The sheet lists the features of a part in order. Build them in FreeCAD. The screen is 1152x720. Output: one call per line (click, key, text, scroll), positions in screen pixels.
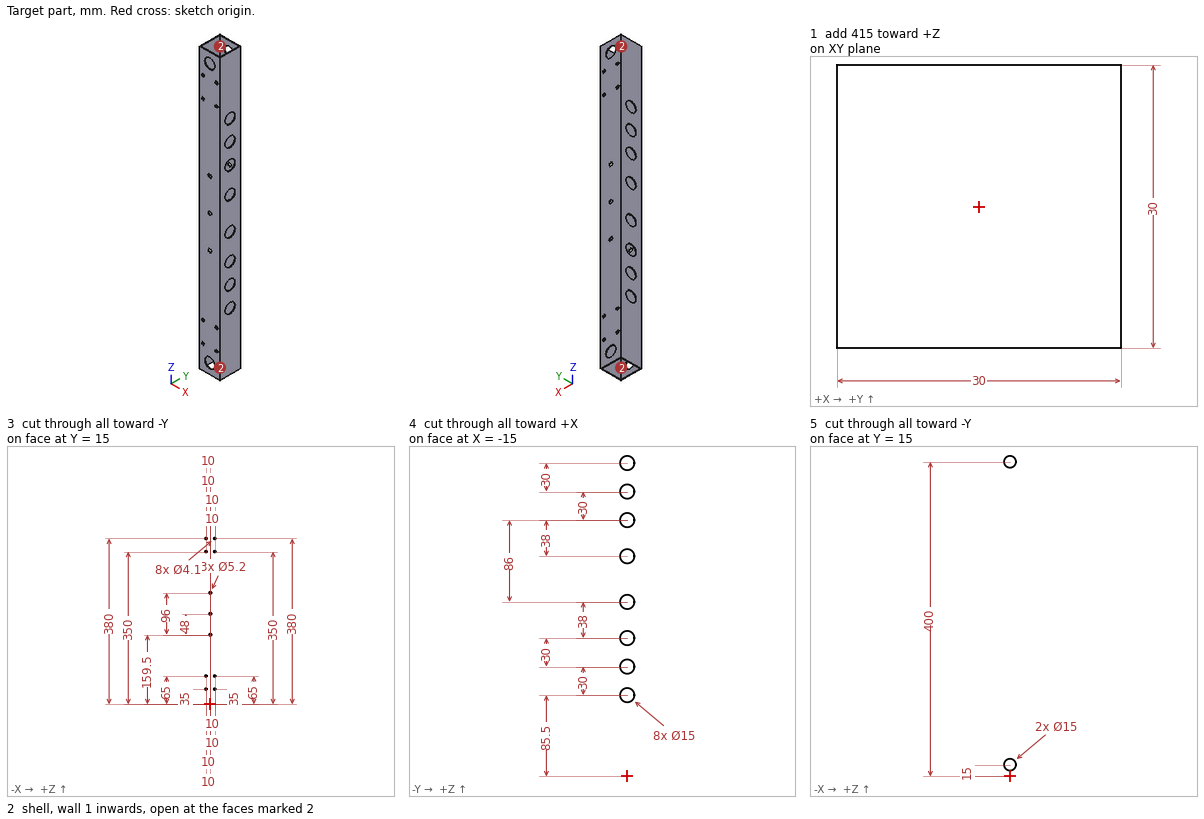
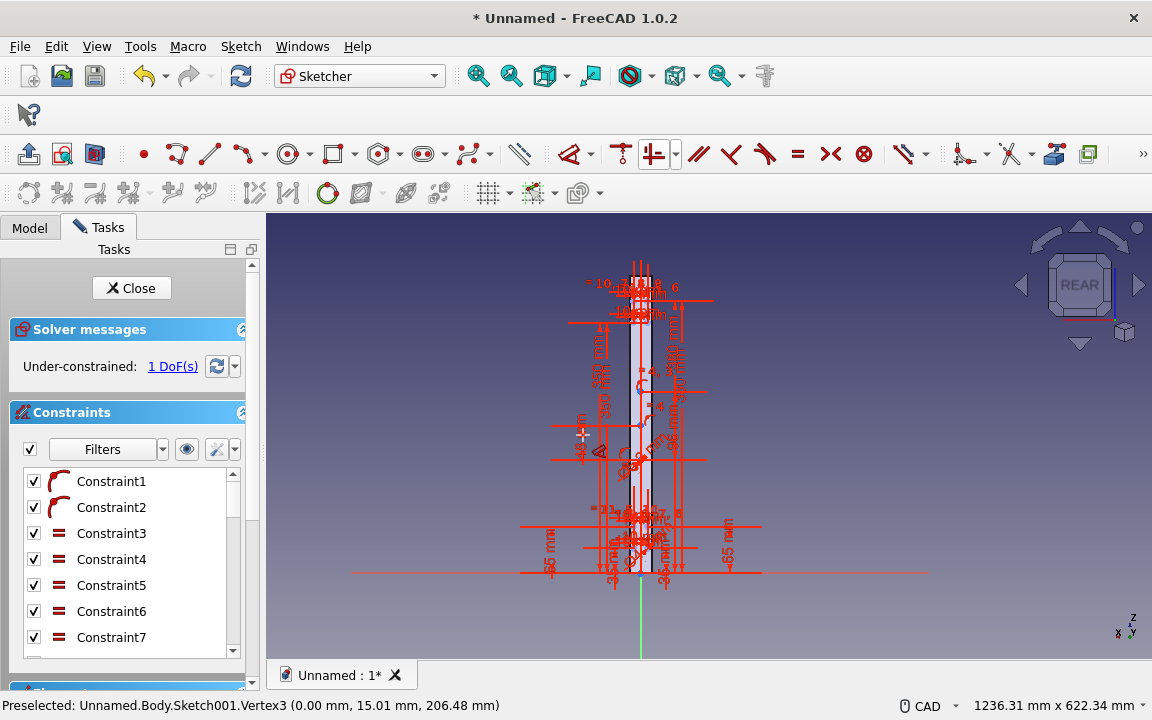
click(641, 460)
click(675, 491)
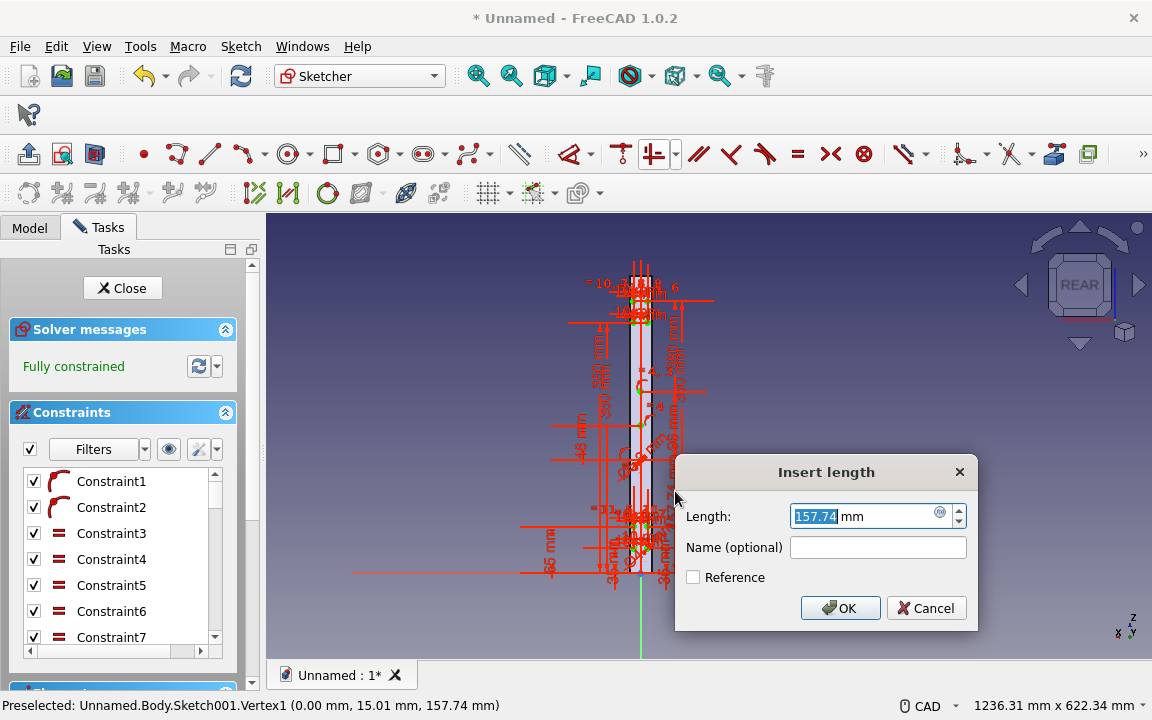
text(159.5)
key(Return)
key(Escape)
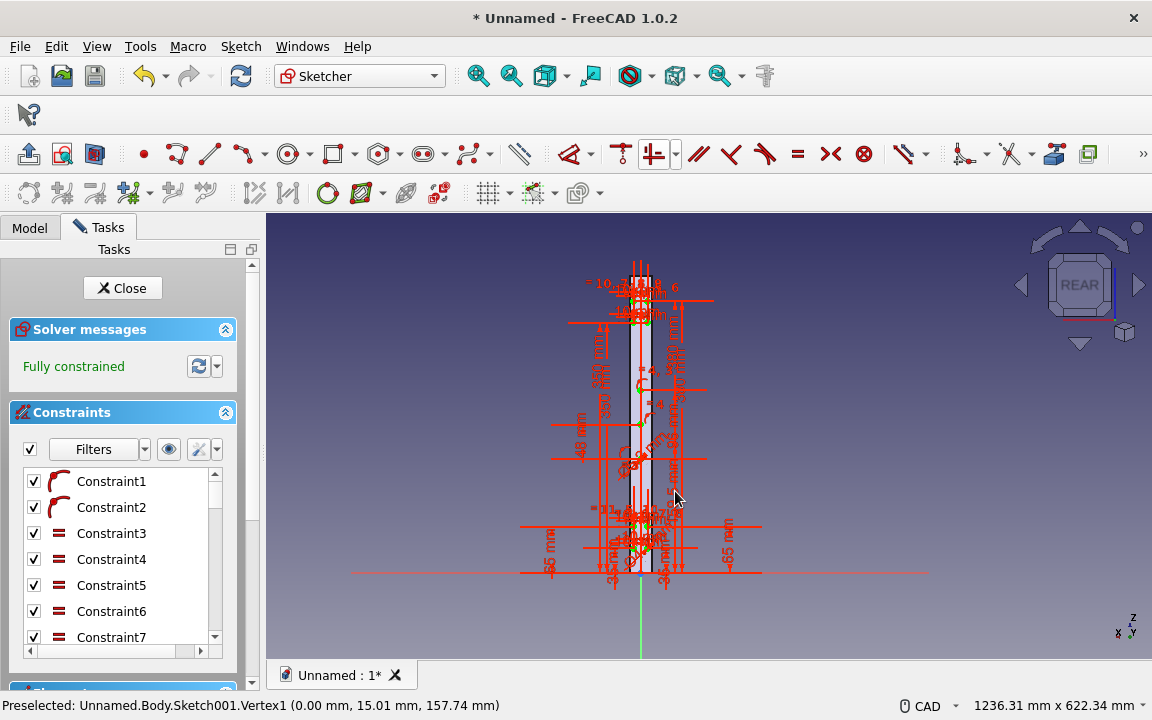
click(123, 288)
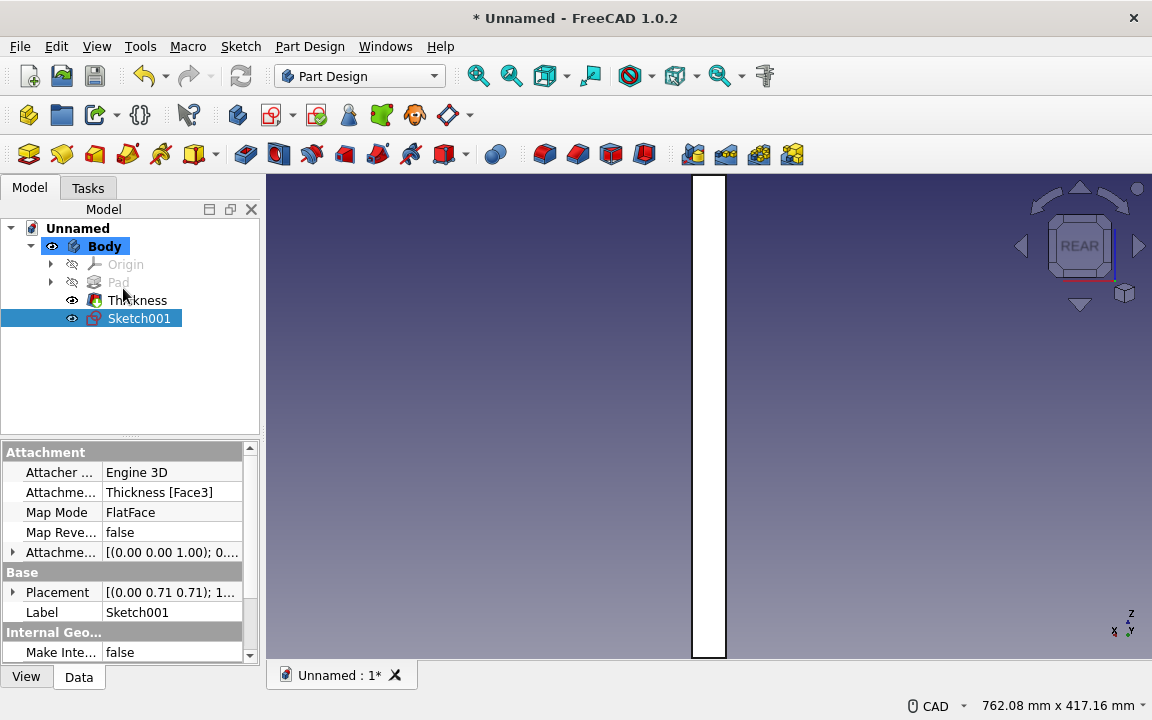
click(246, 154)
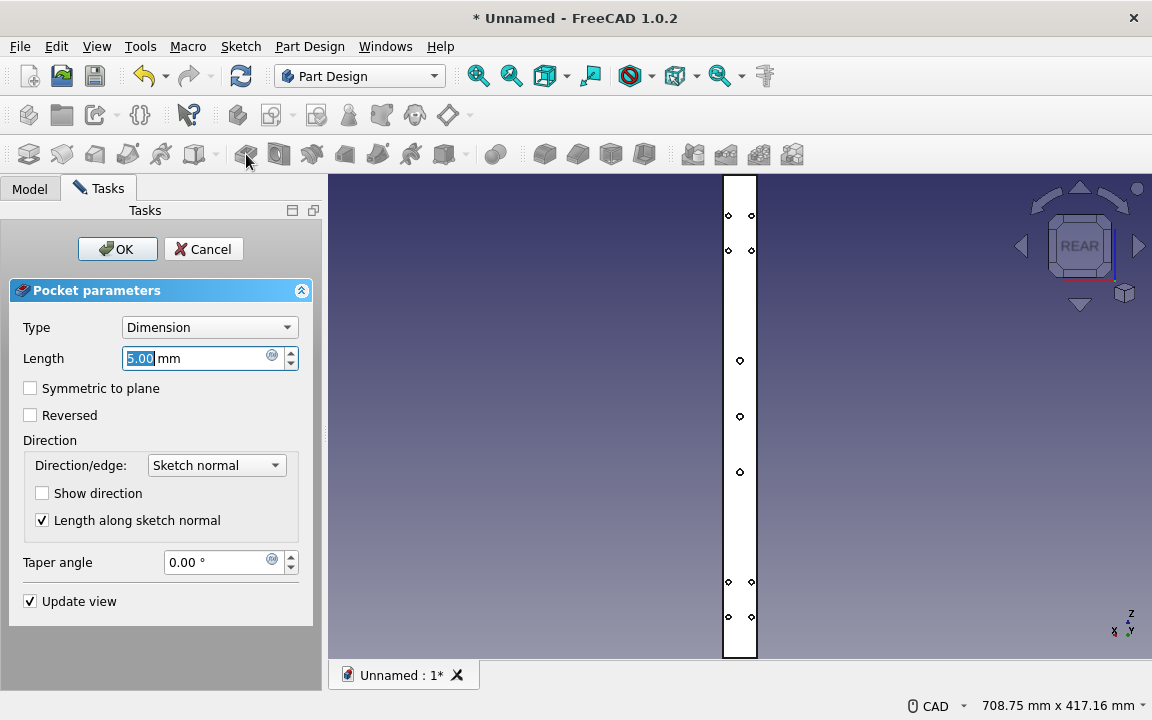
click(210, 328)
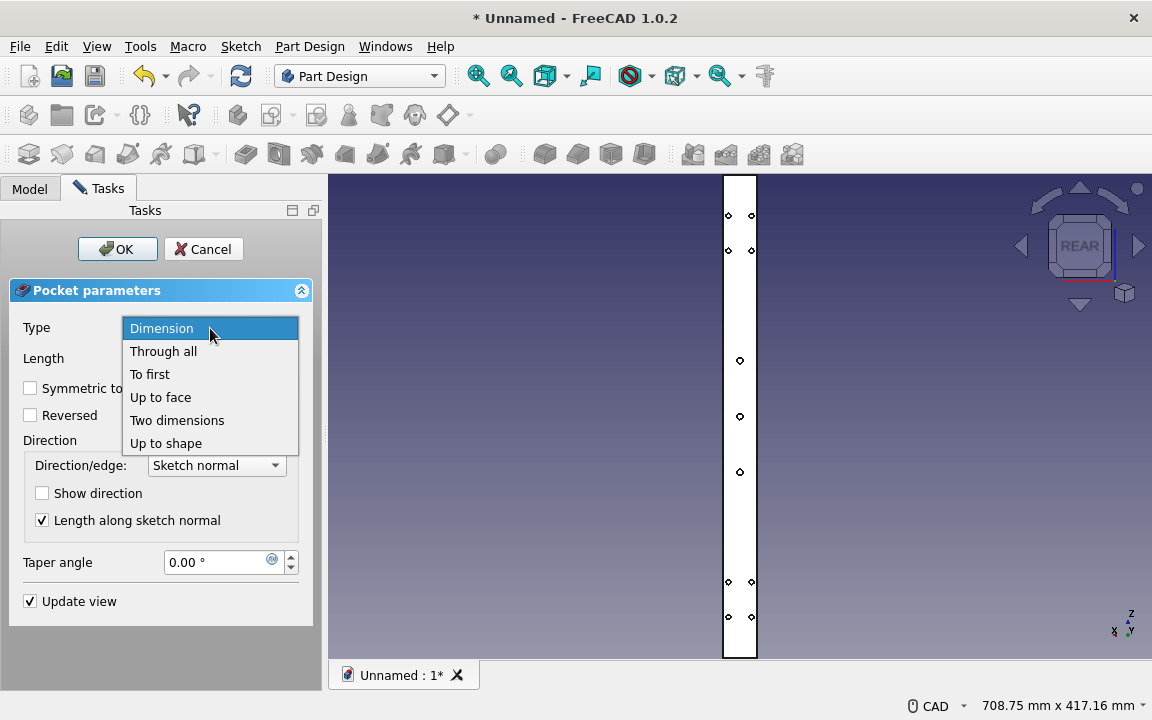
click(208, 352)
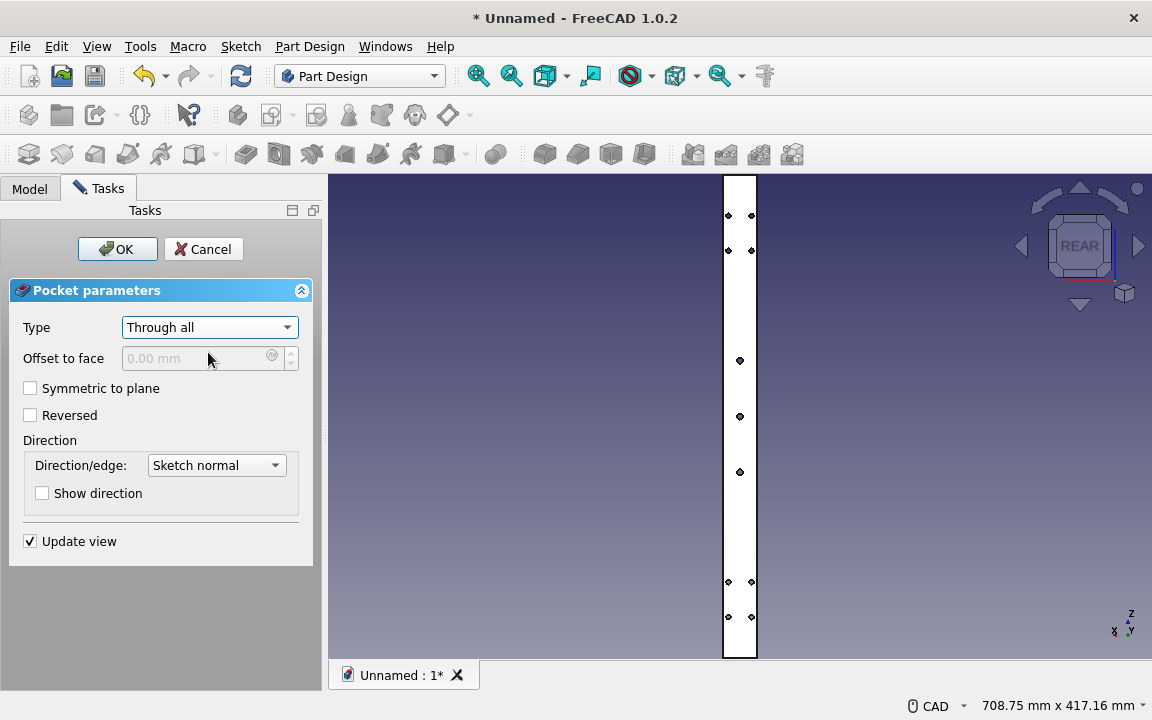
click(118, 249)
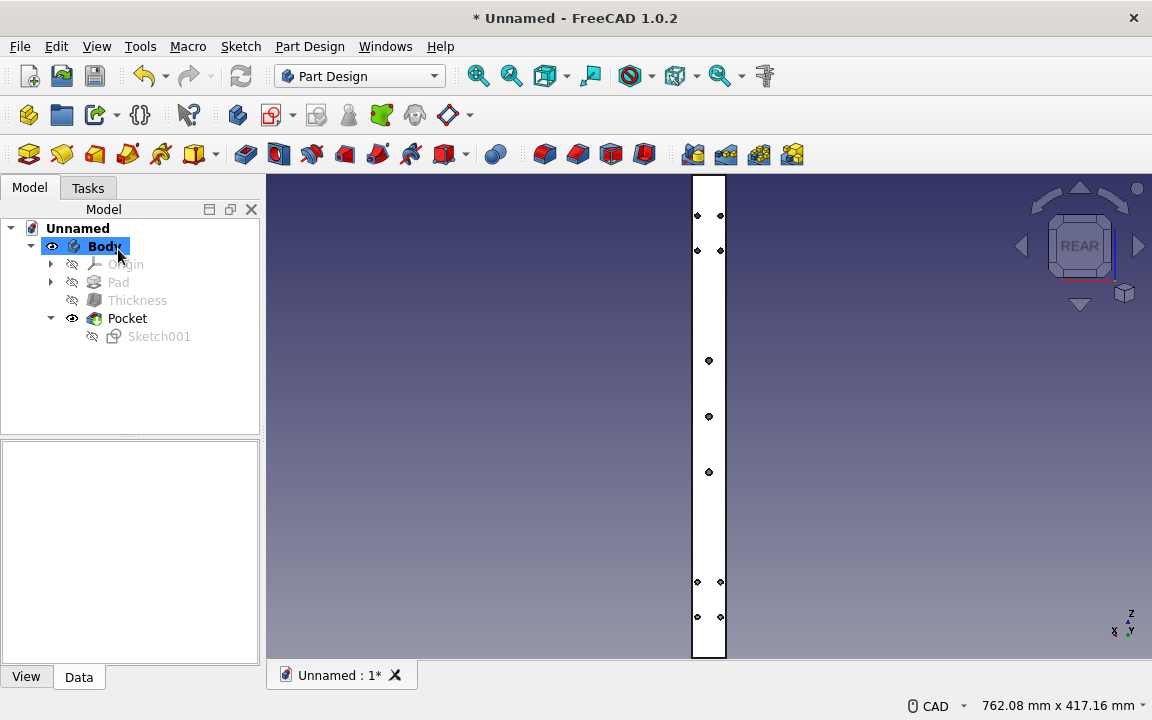
key(6)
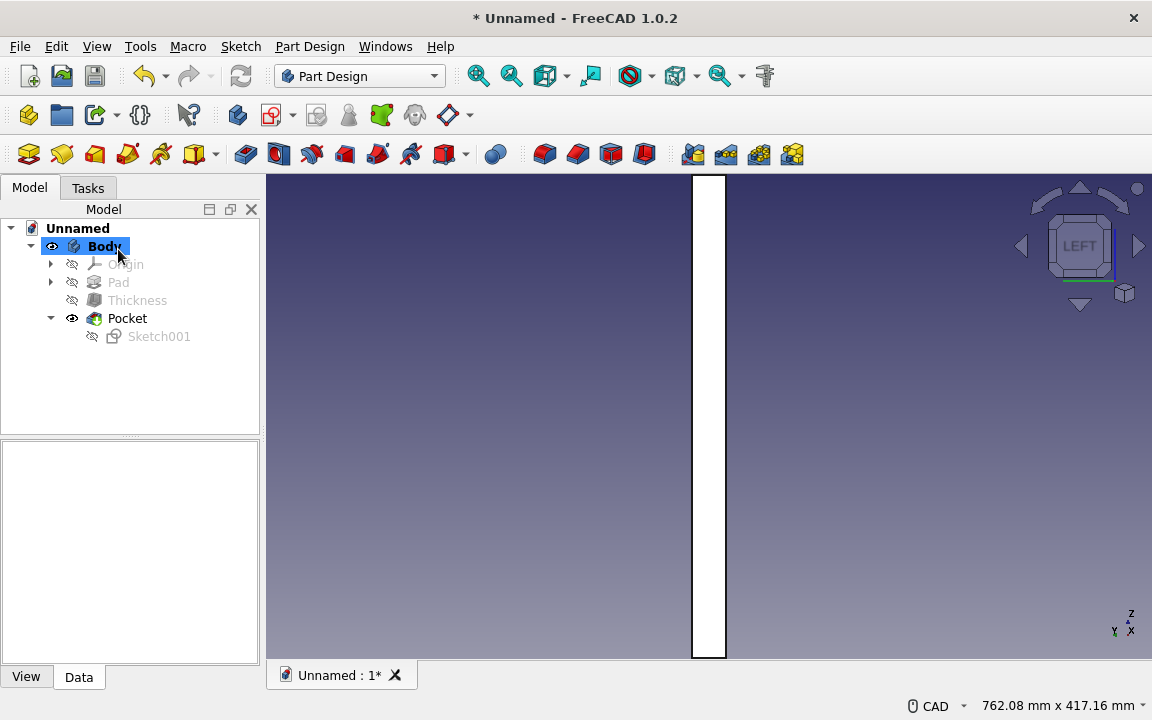
click(709, 209)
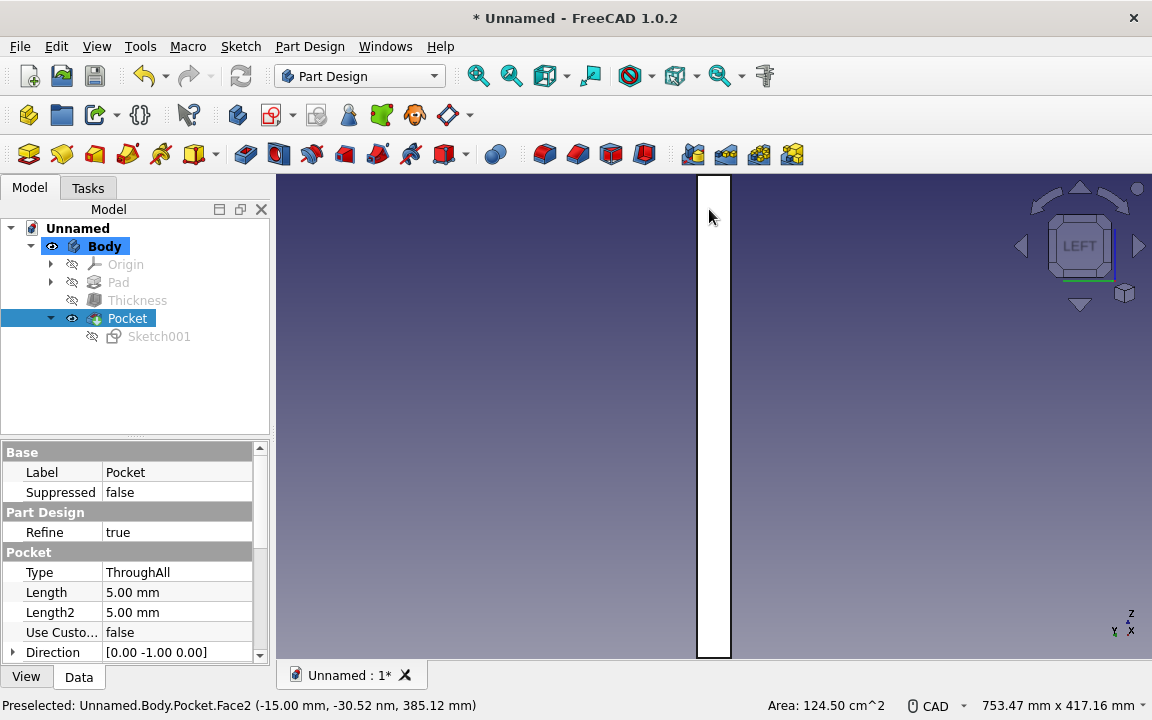
click(270, 116)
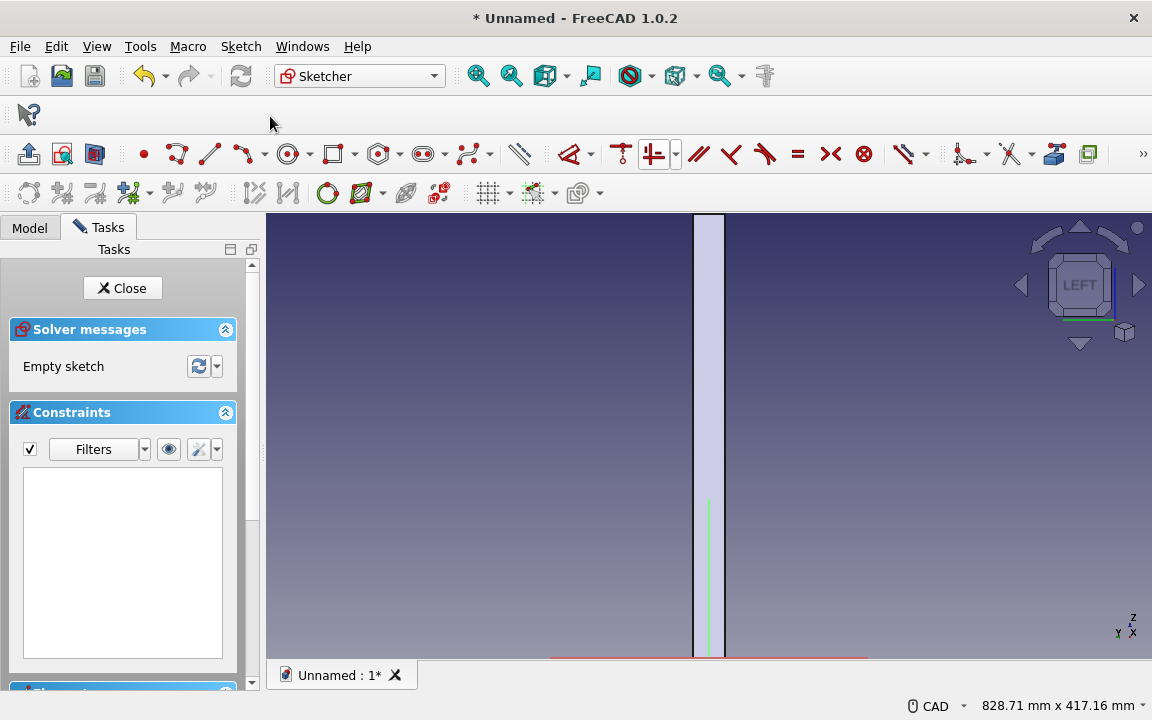
scroll(331, 248, down, 1)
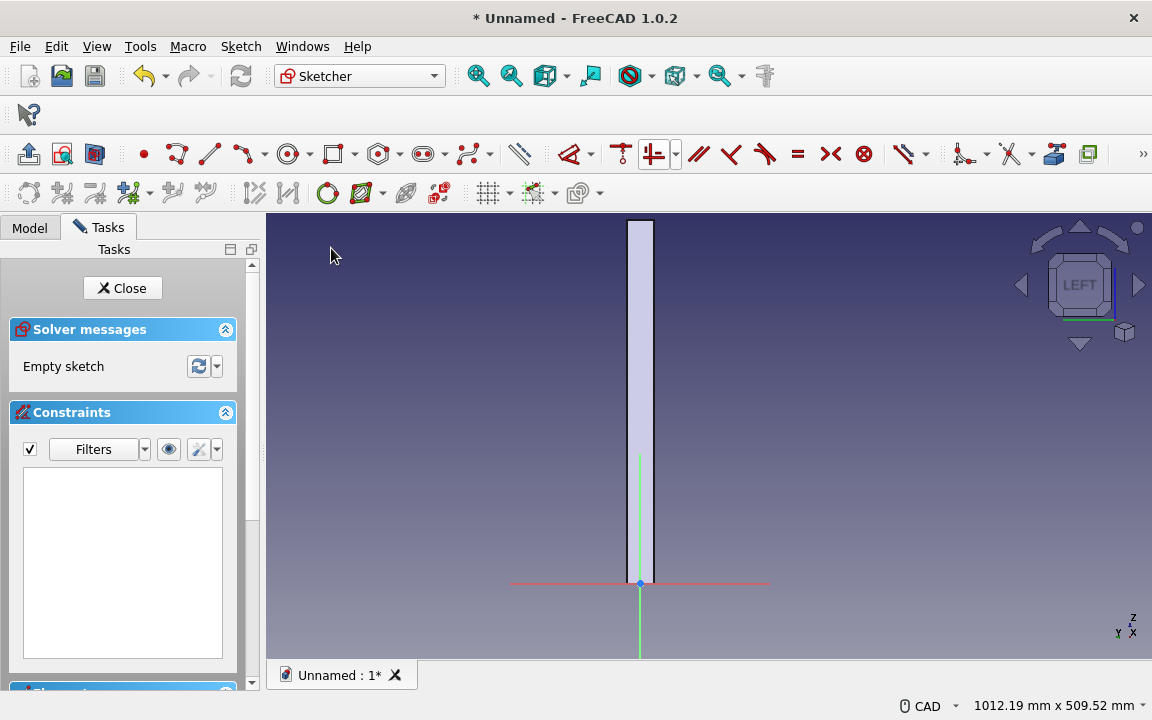
click(288, 154)